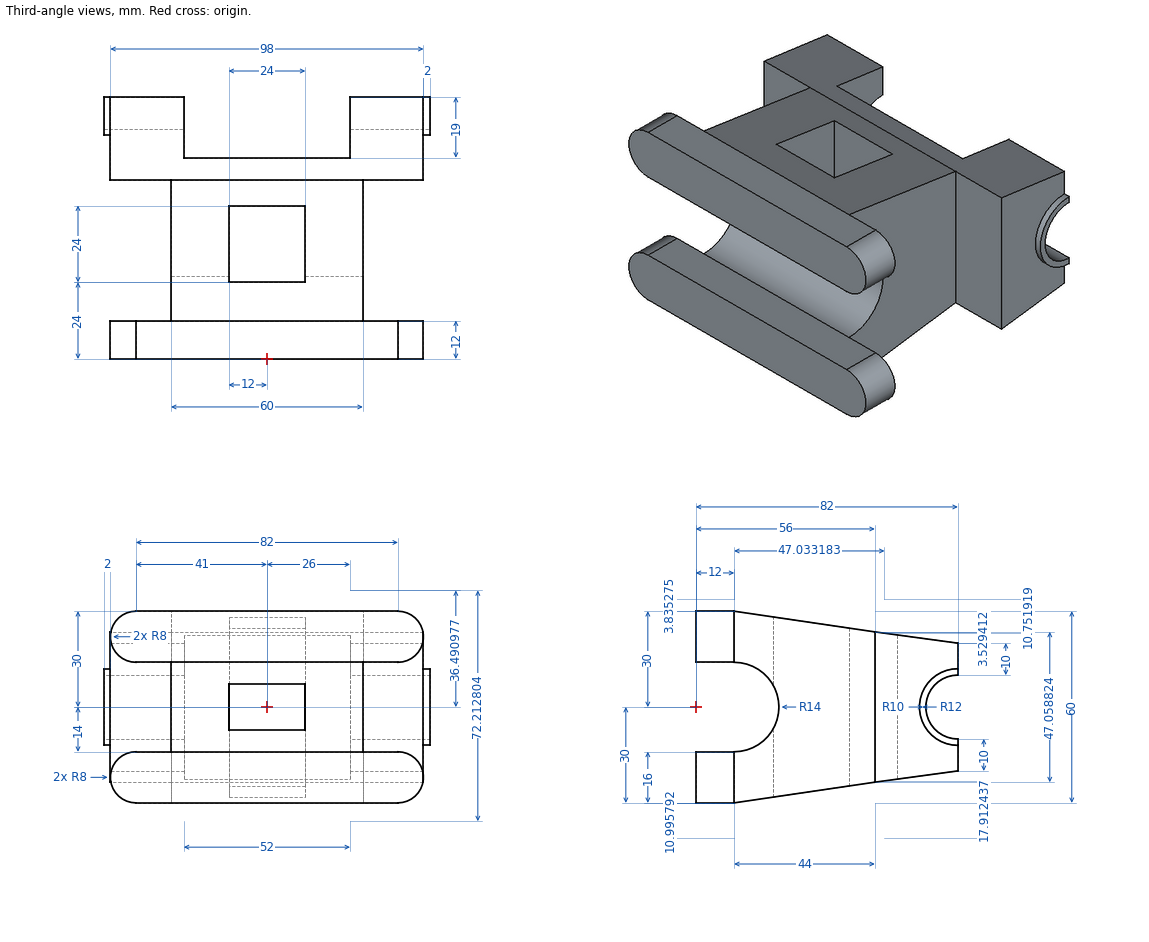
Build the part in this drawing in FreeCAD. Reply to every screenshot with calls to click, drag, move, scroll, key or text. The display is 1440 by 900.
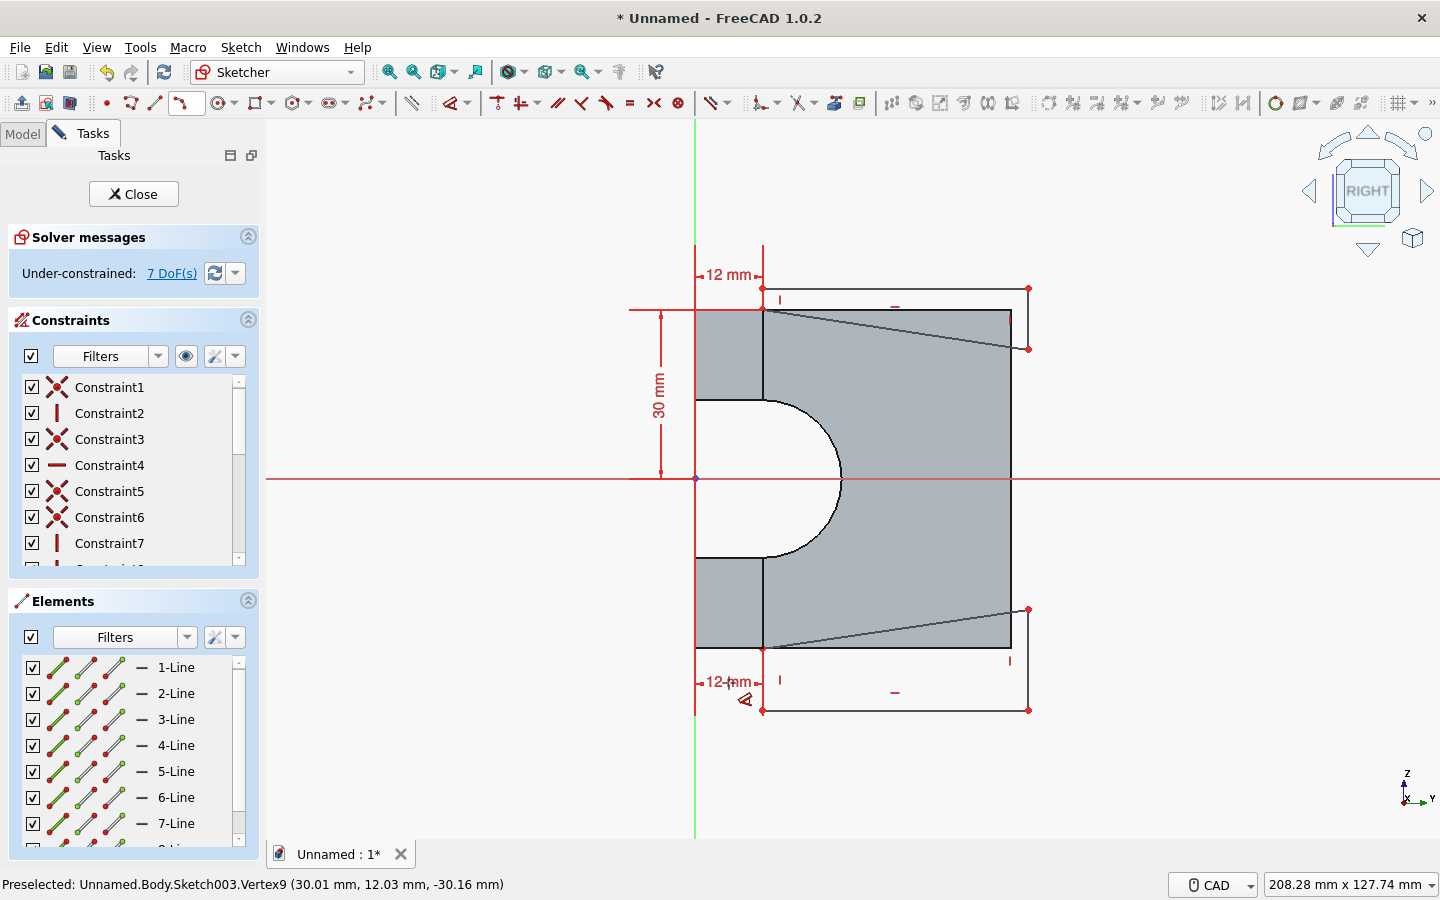
click(763, 649)
click(661, 564)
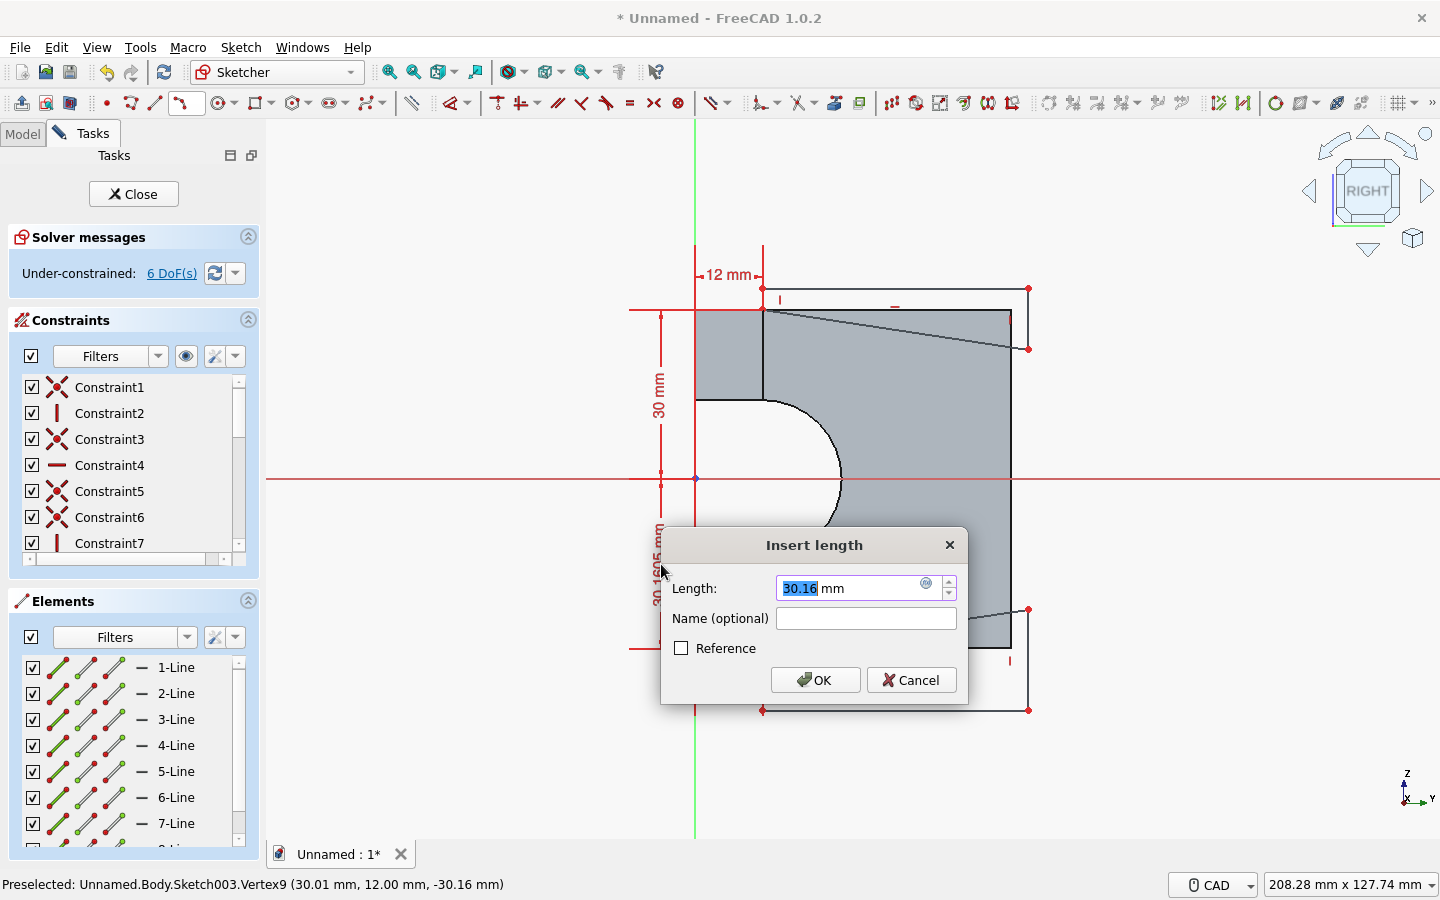
text(30)
key(Return)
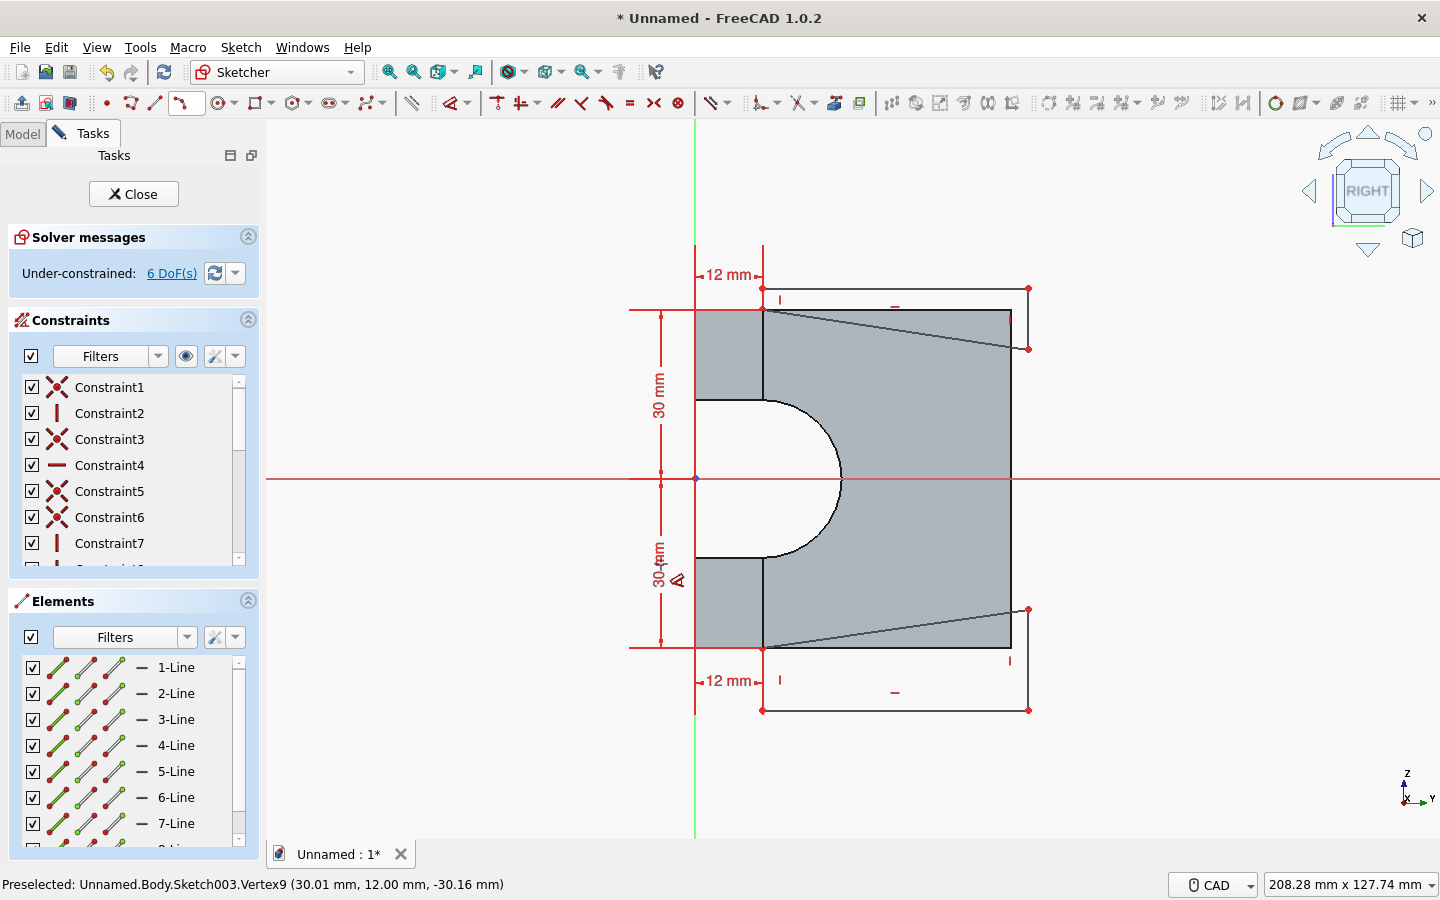
scroll(763, 299, up, 4)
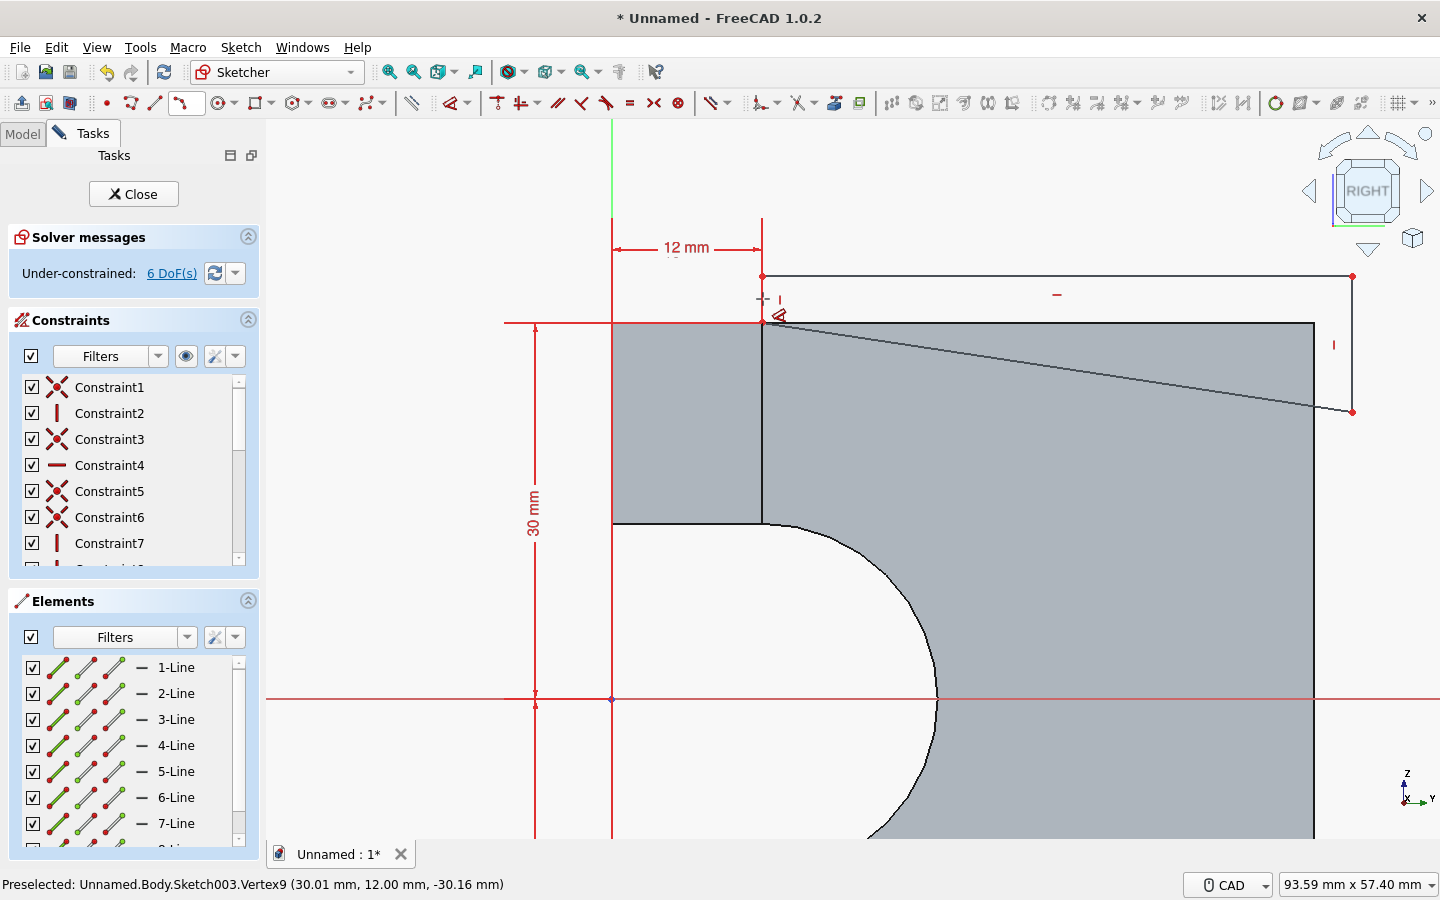
click(762, 300)
click(728, 300)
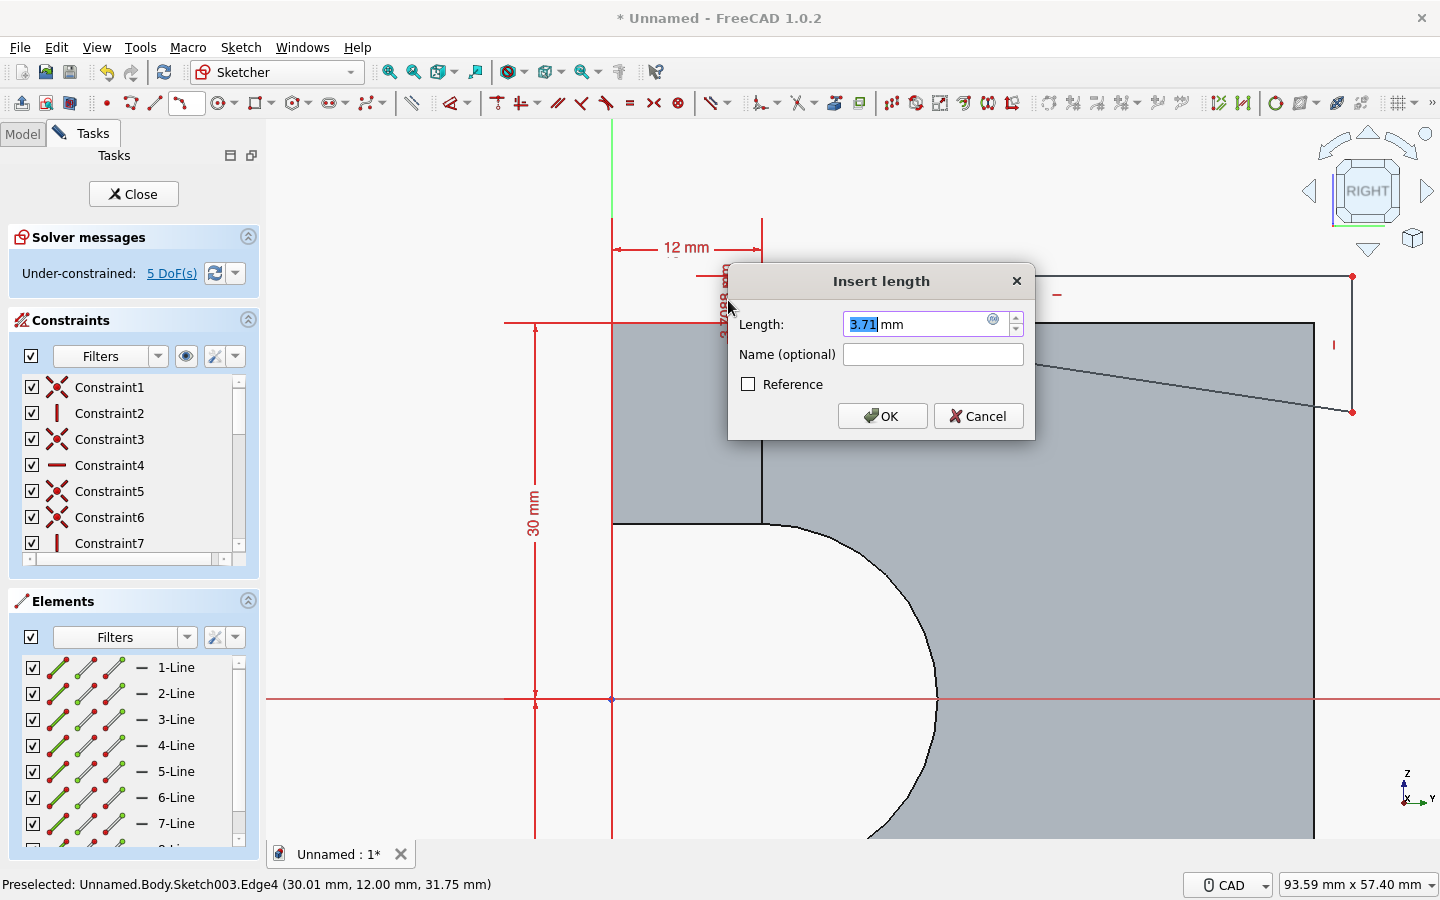
text(3.835275)
key(Return)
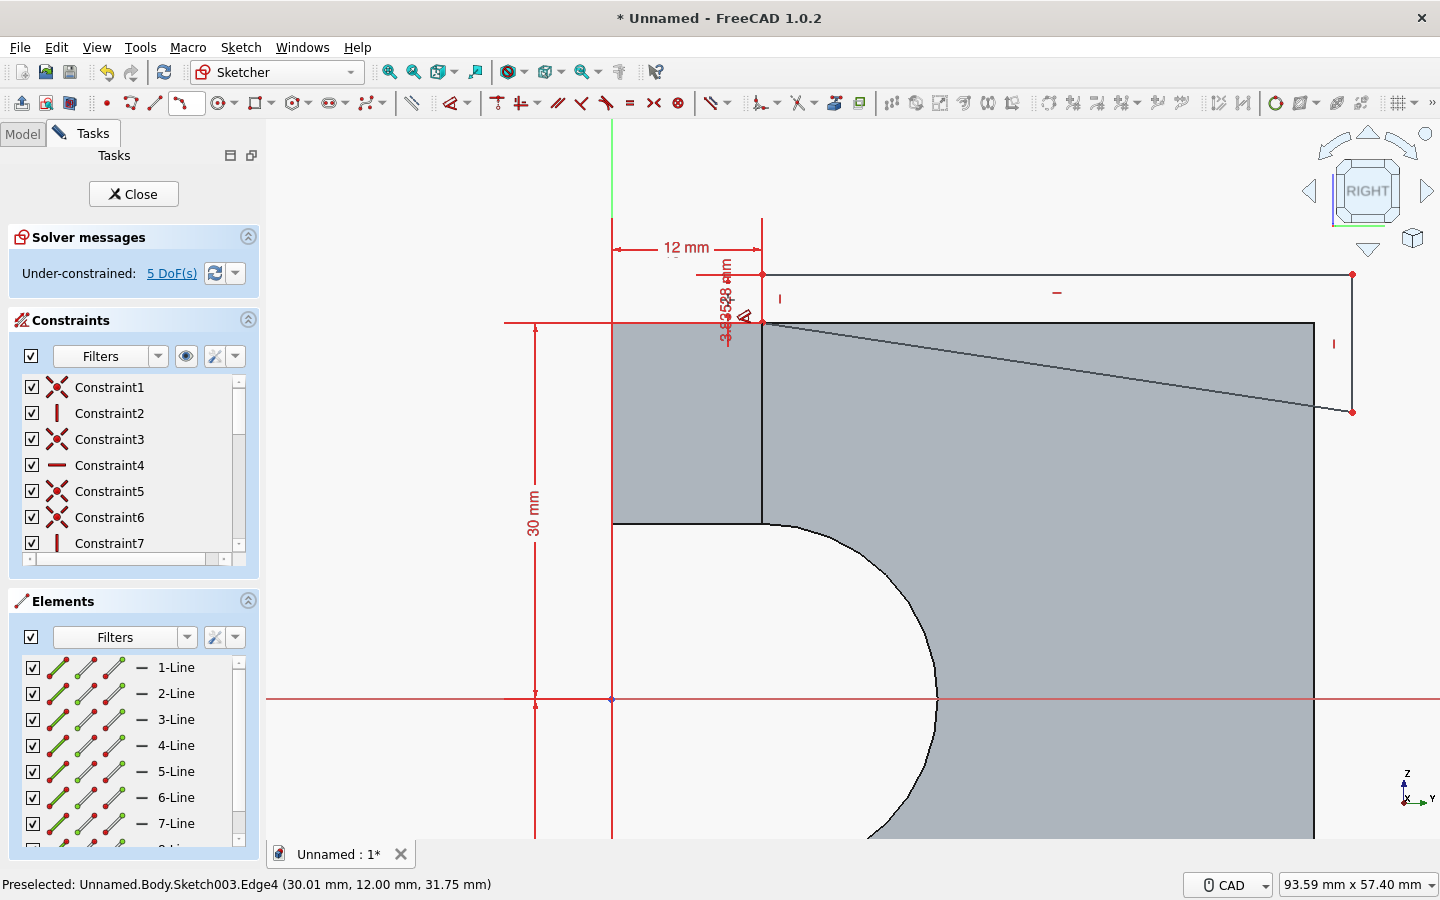
scroll(545, 156, down, 3)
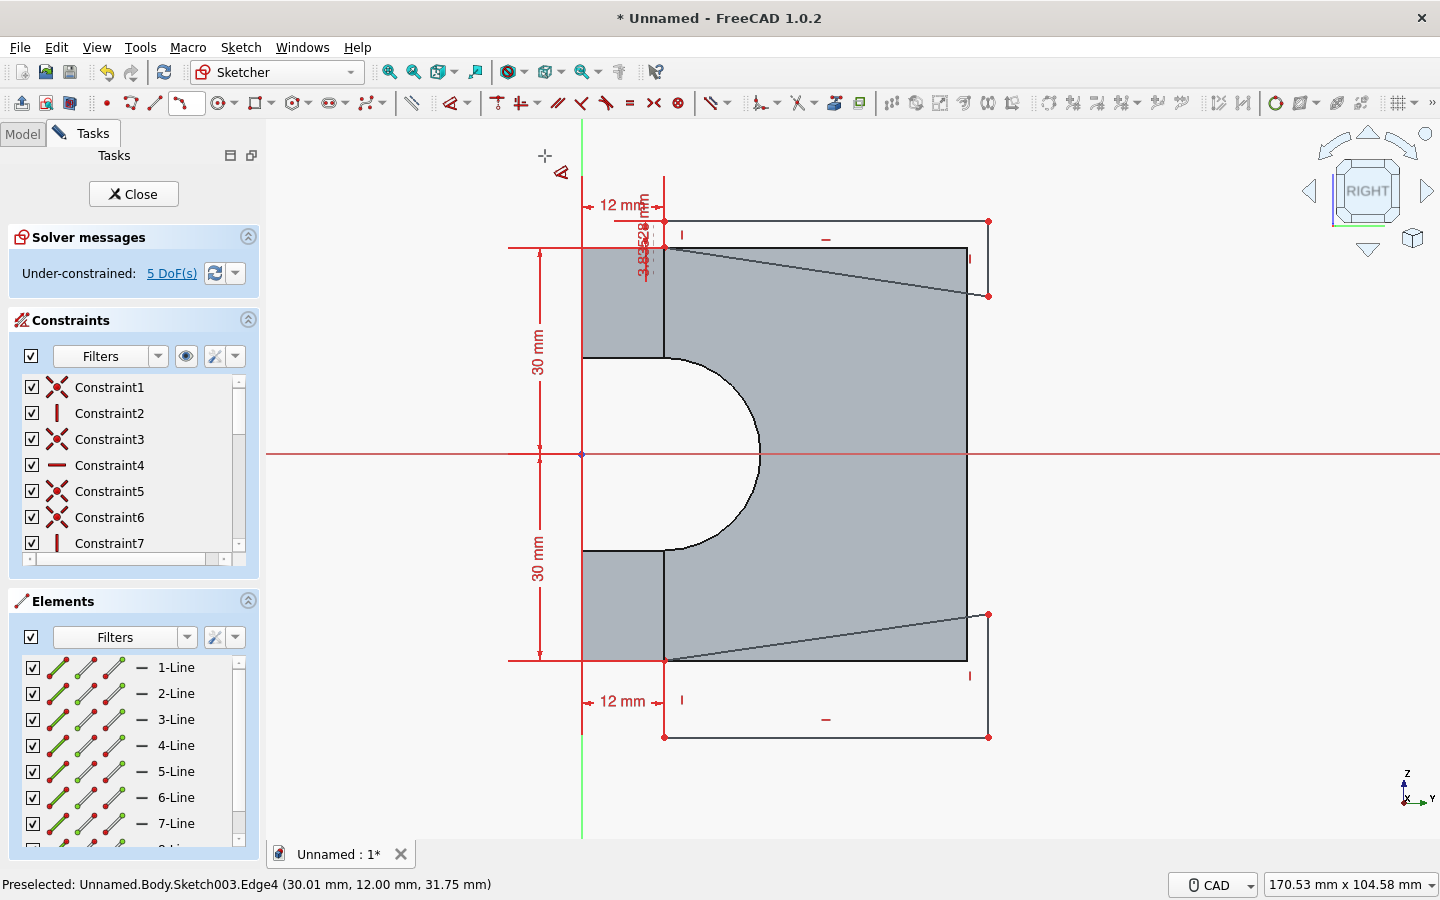
click(988, 274)
click(1022, 259)